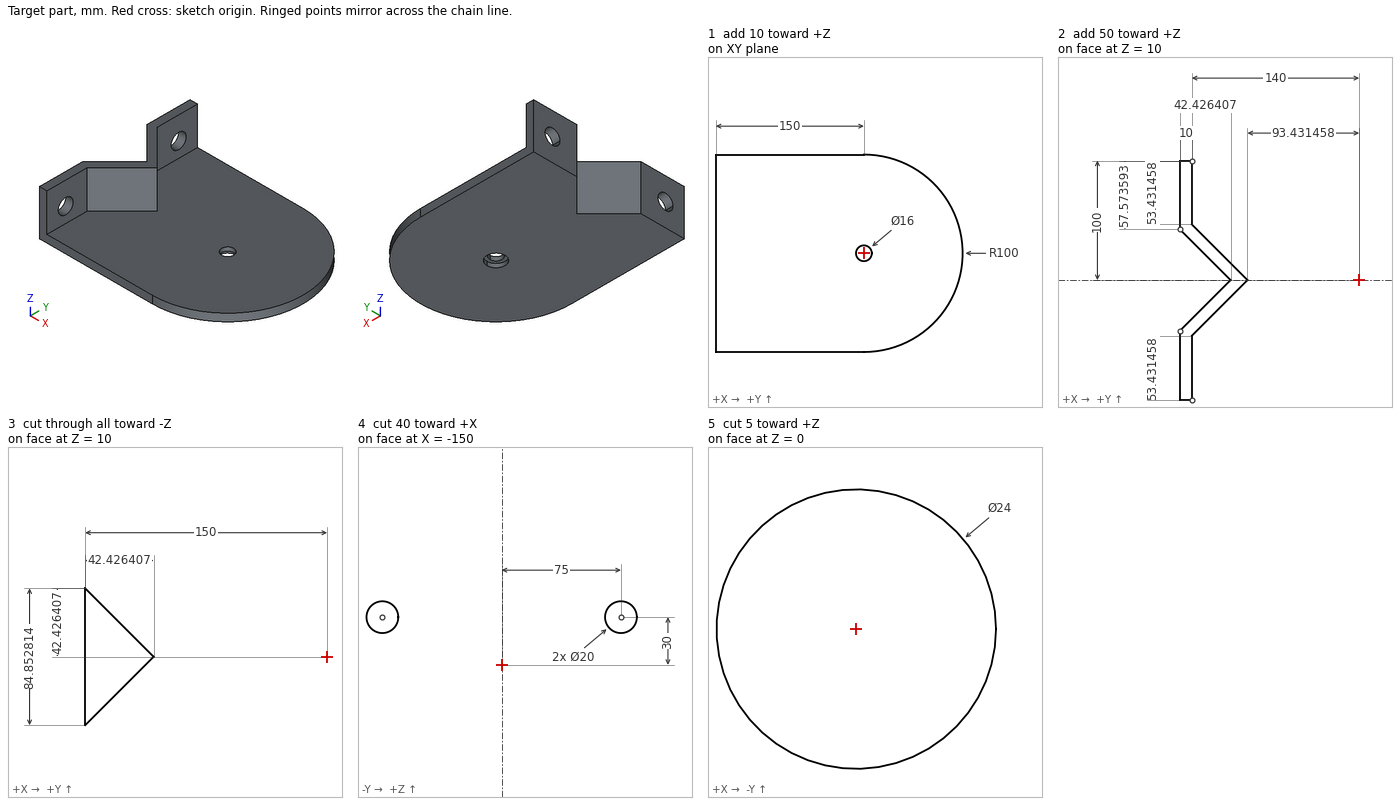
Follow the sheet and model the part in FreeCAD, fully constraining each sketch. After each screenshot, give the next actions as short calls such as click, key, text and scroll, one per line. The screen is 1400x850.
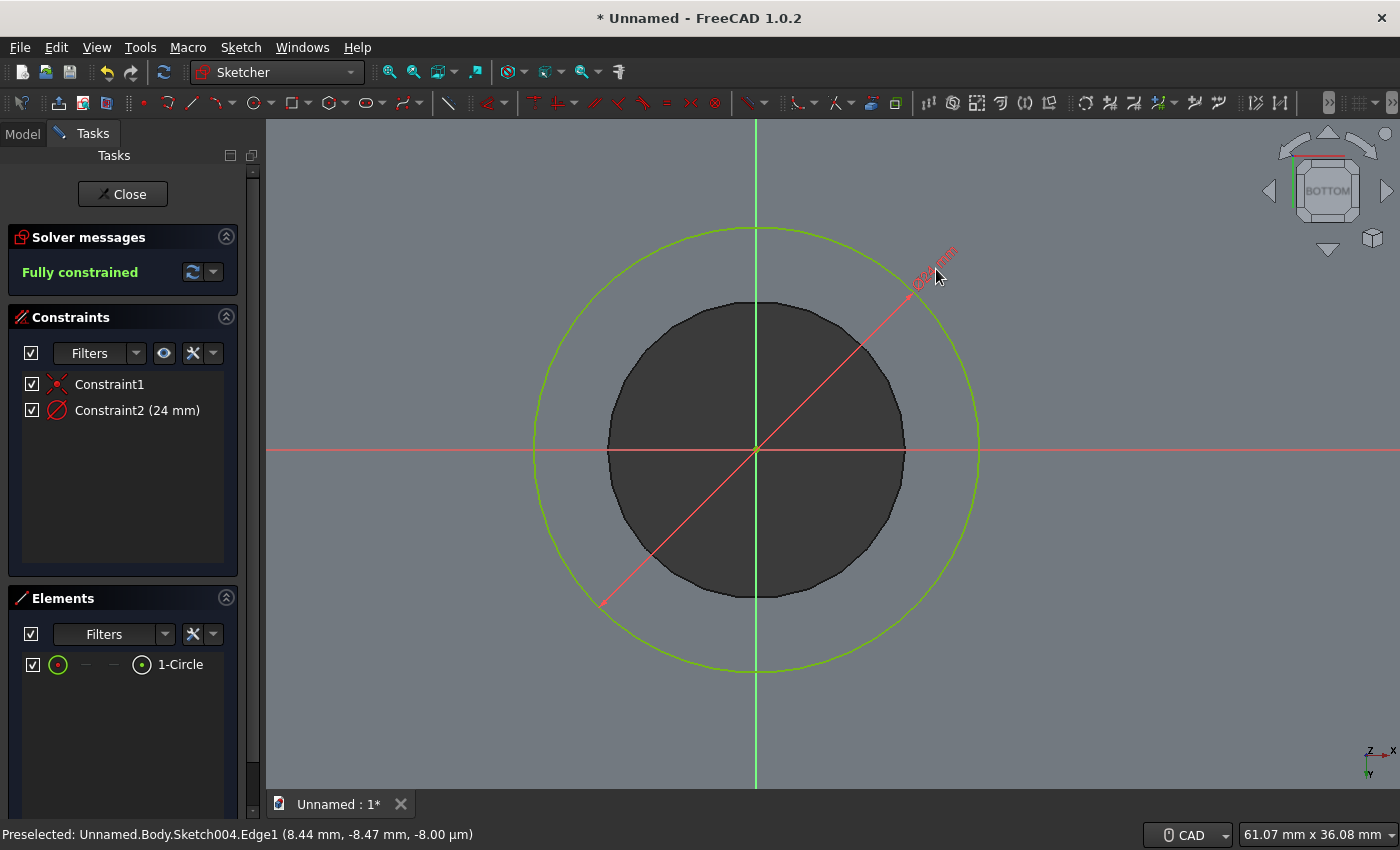
click(123, 194)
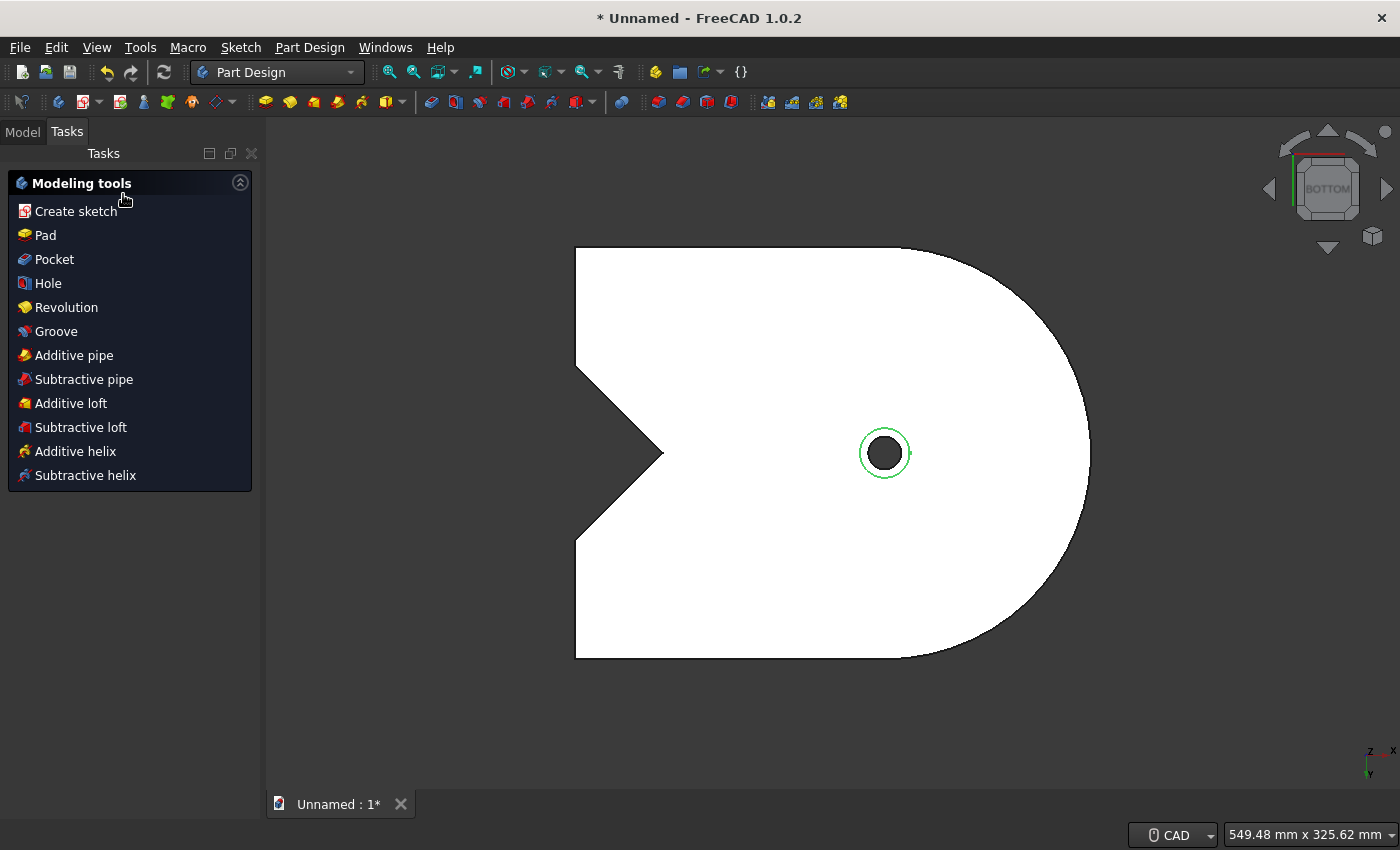
click(432, 102)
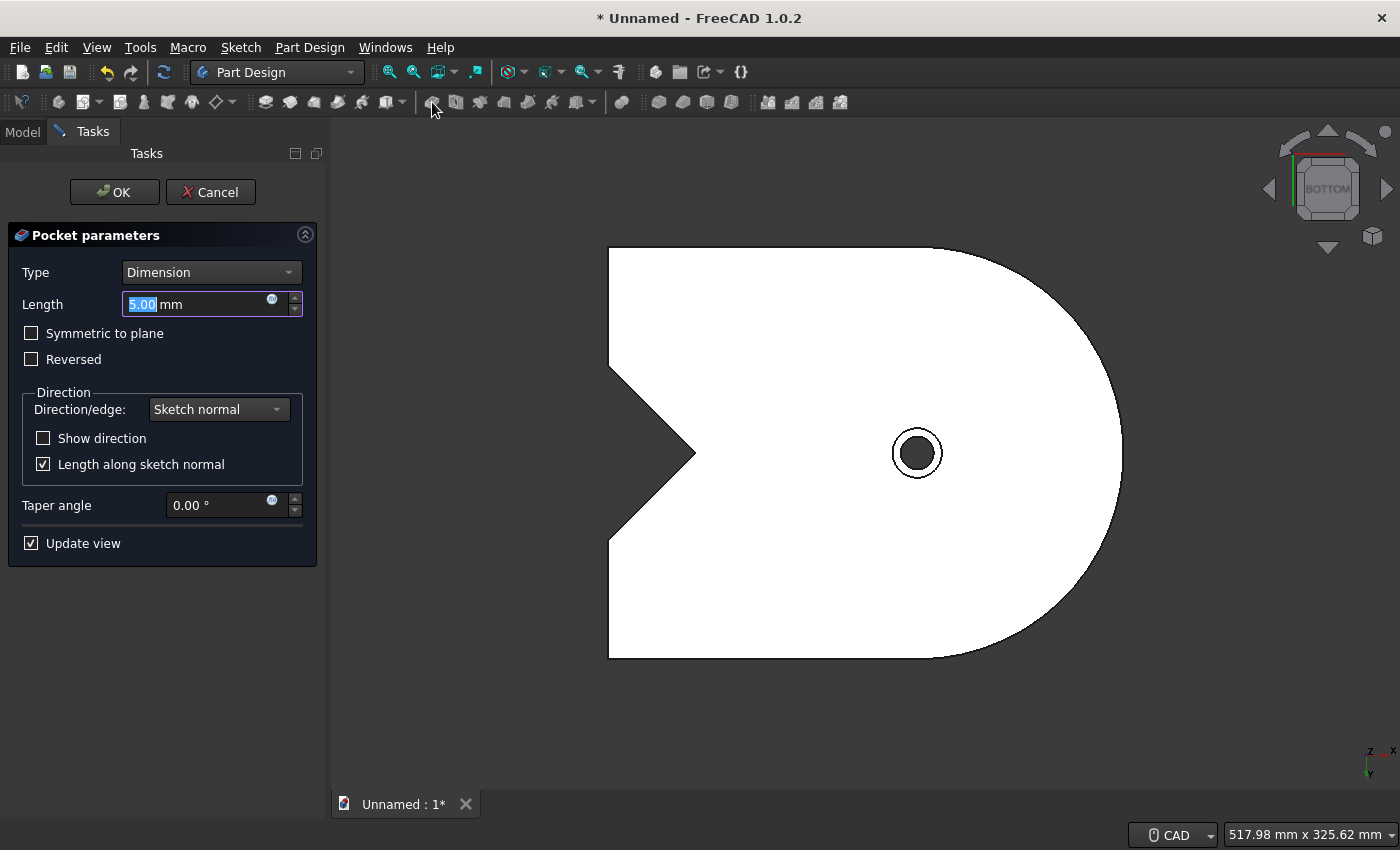
text(5)
key(Tab)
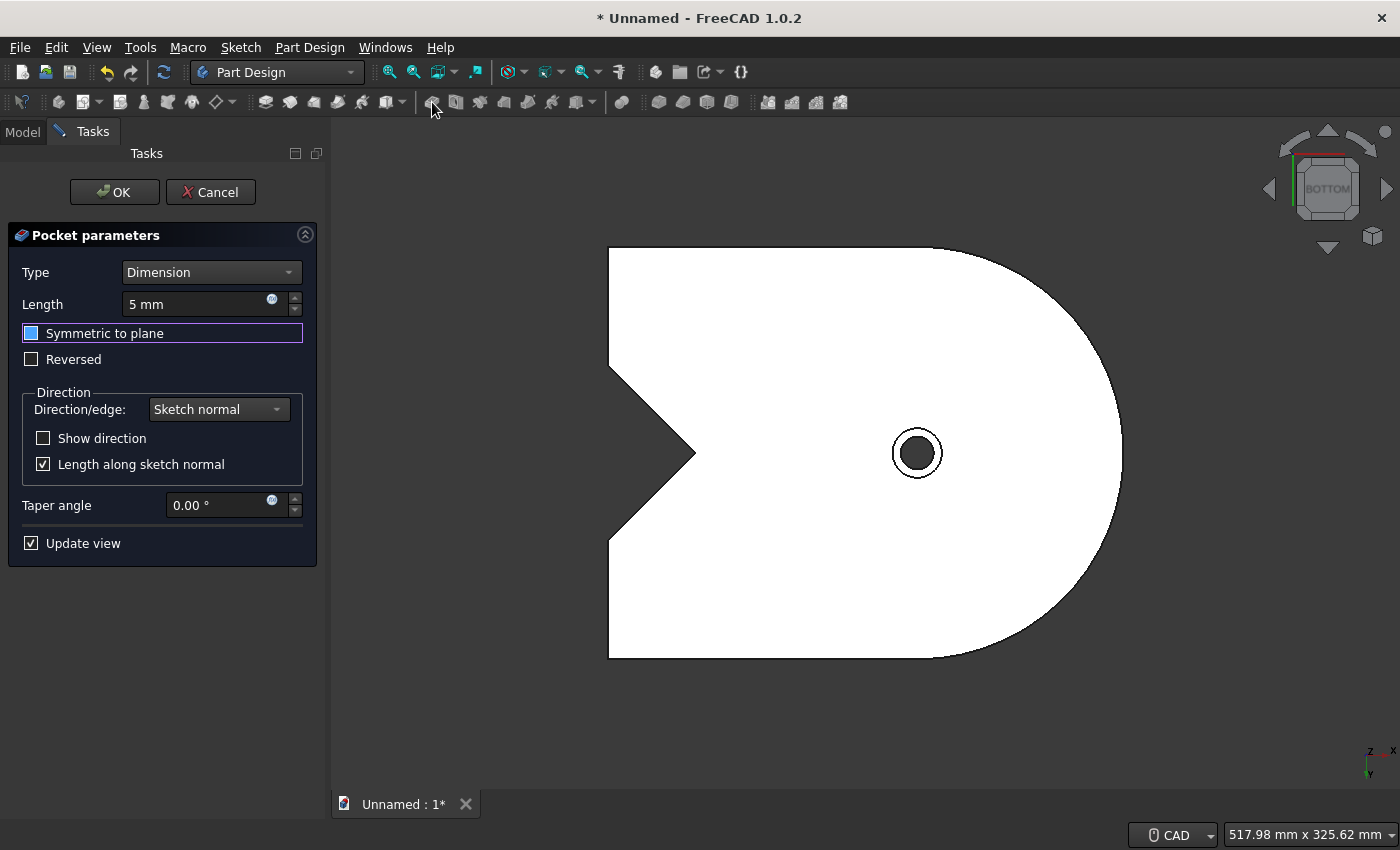
click(115, 192)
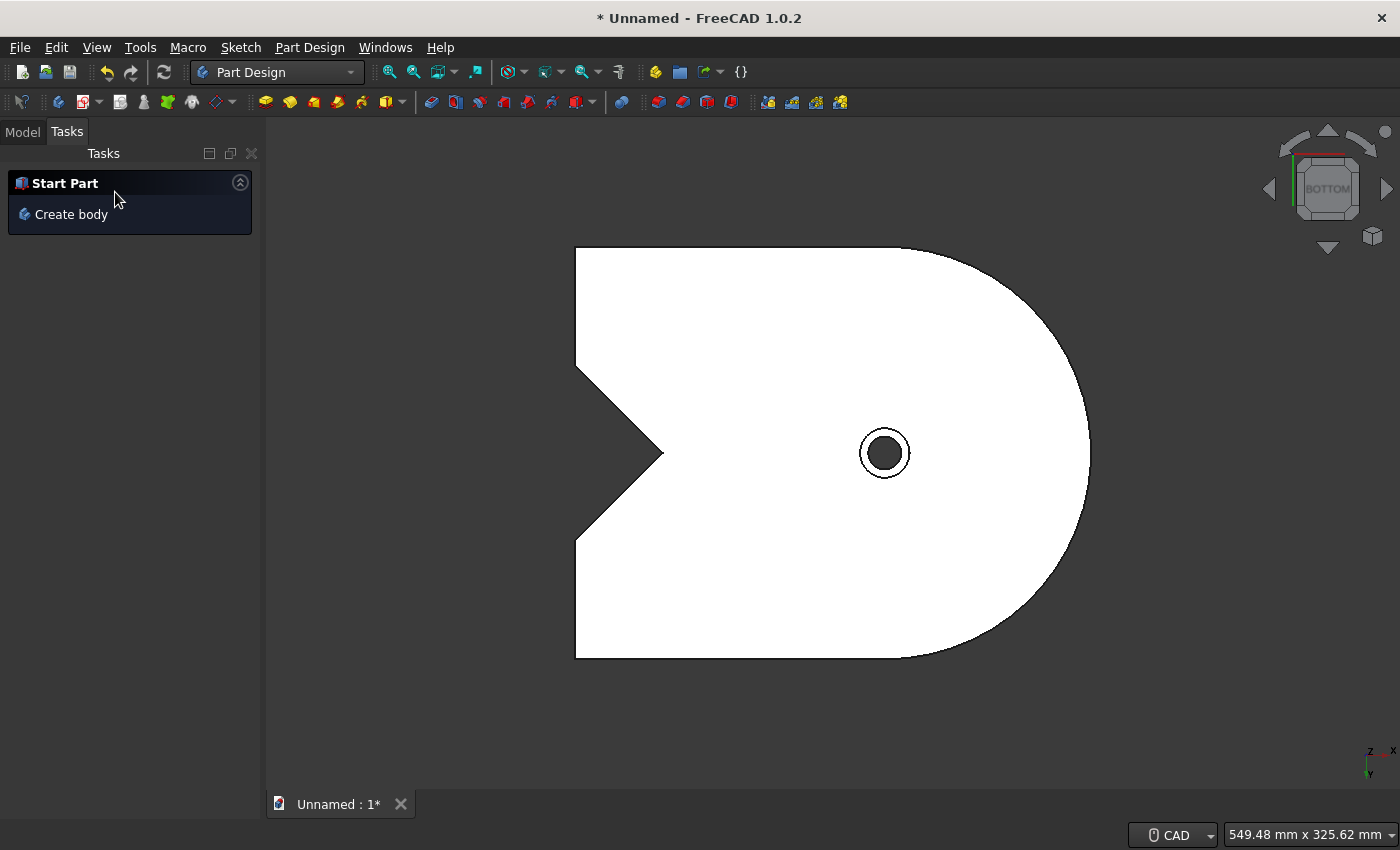
key(0)